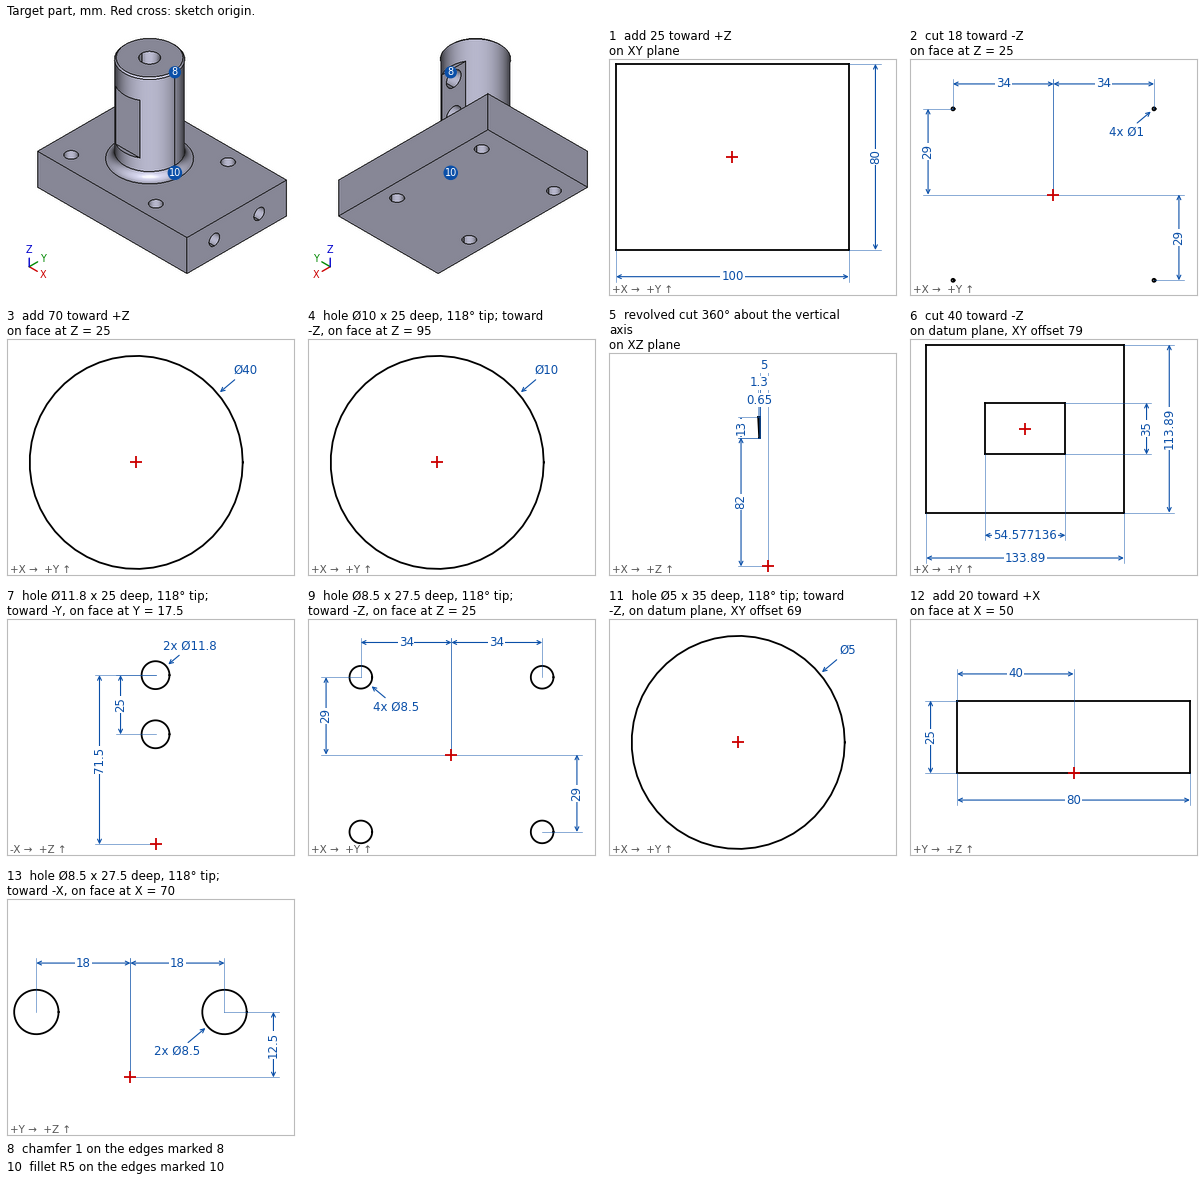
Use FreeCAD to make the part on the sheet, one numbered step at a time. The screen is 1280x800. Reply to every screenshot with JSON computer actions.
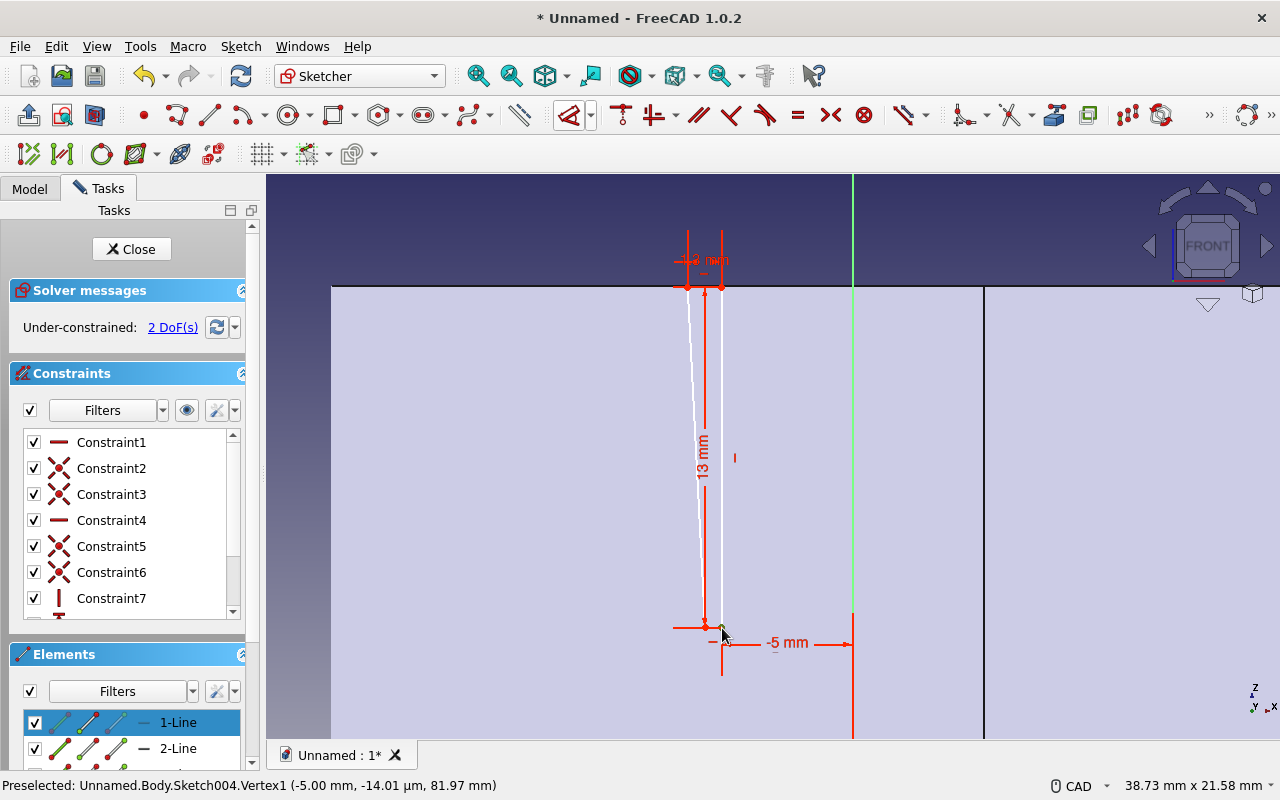
{"action": "key", "text": "i"}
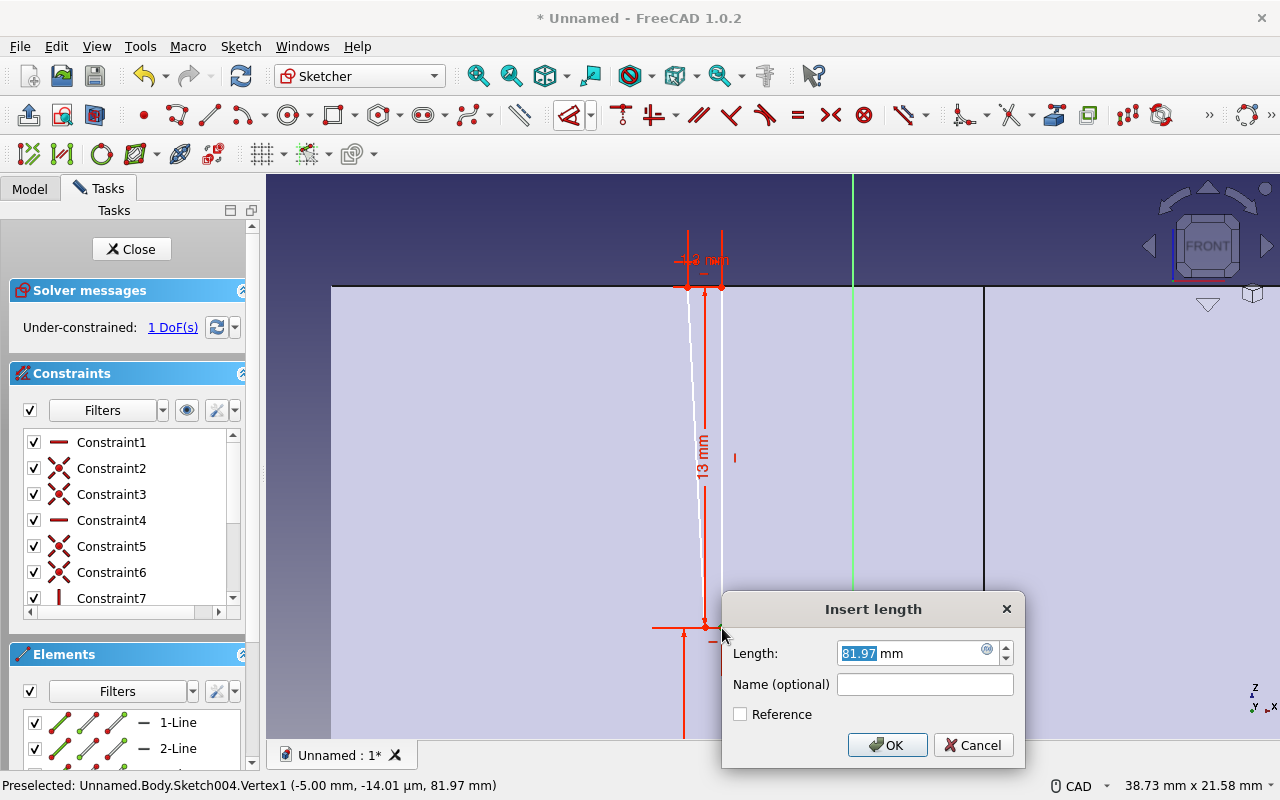
{"action": "type", "text": "82"}
{"action": "key", "text": "Return"}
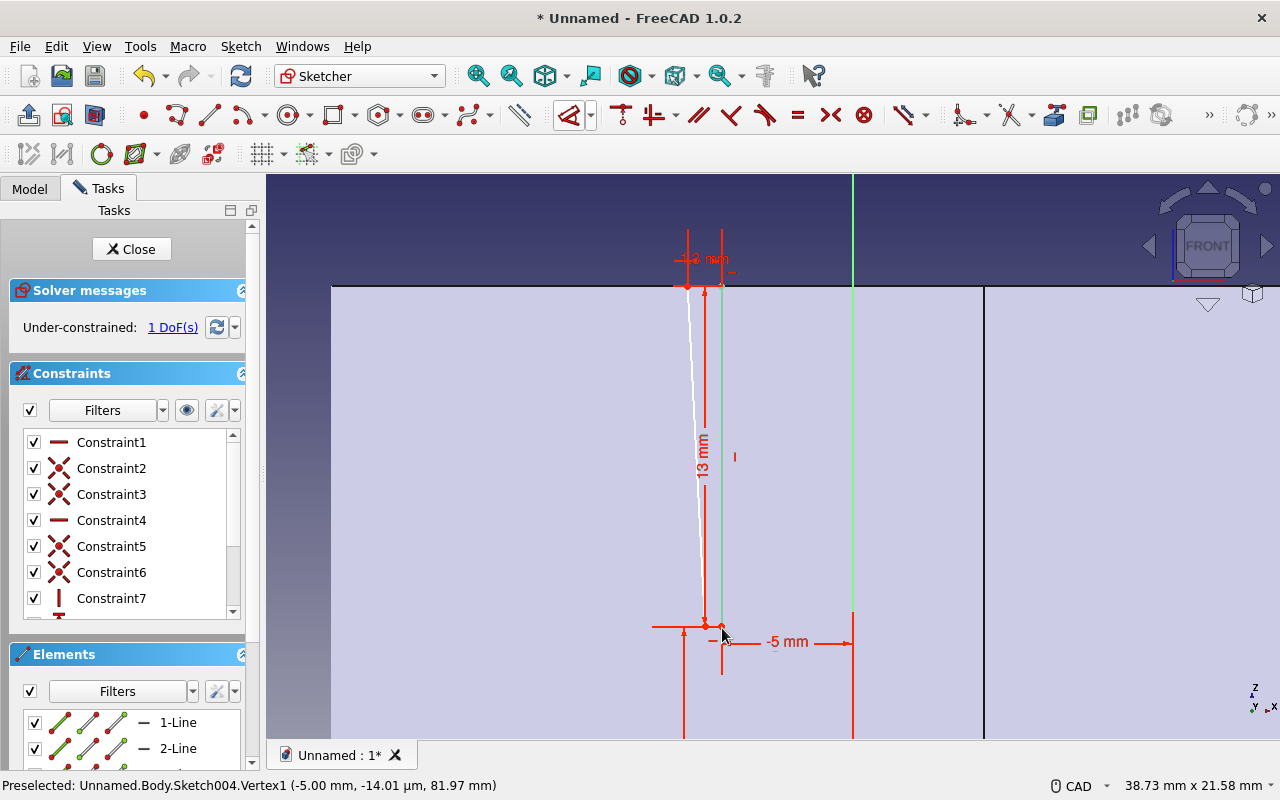
{"action": "scroll", "coordinate": [713, 627], "scroll_direction": "up", "scroll_amount": 5}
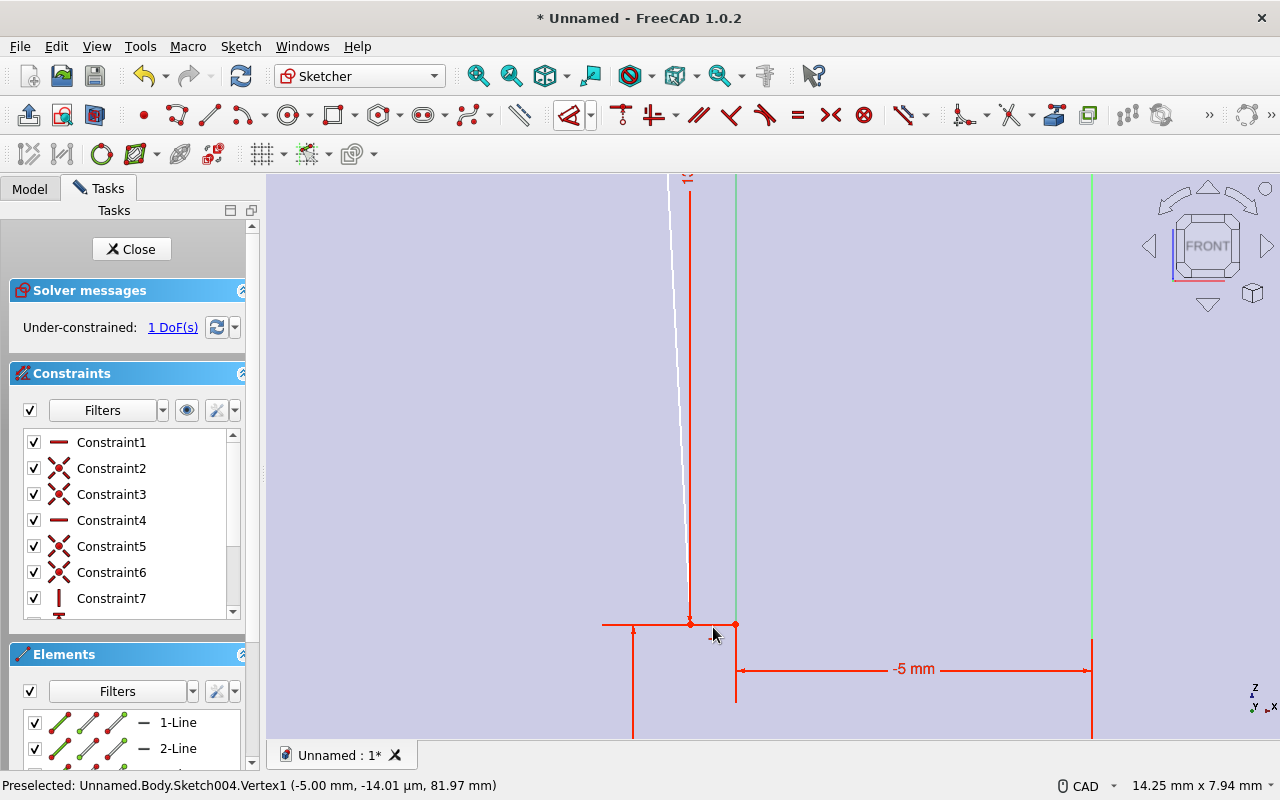
{"action": "left_click", "coordinate": [713, 625]}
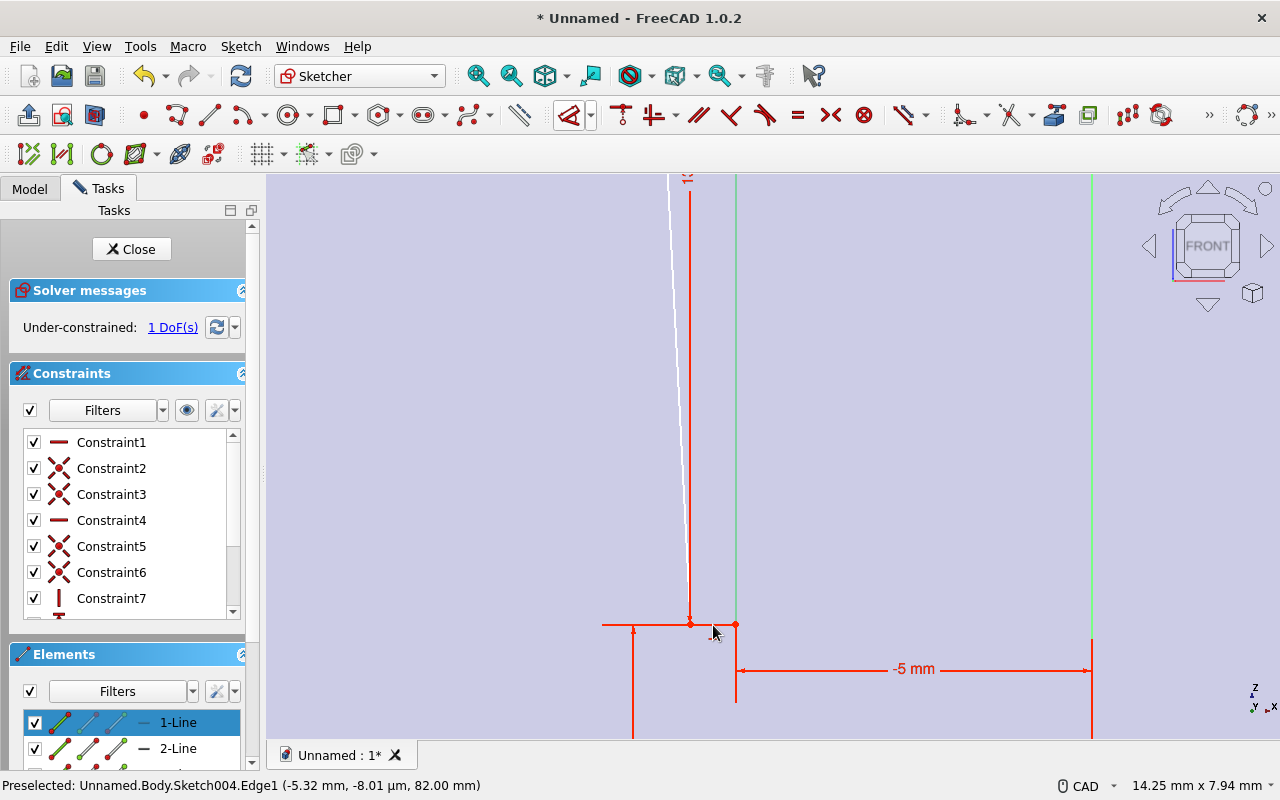
{"action": "left_click", "coordinate": [590, 116]}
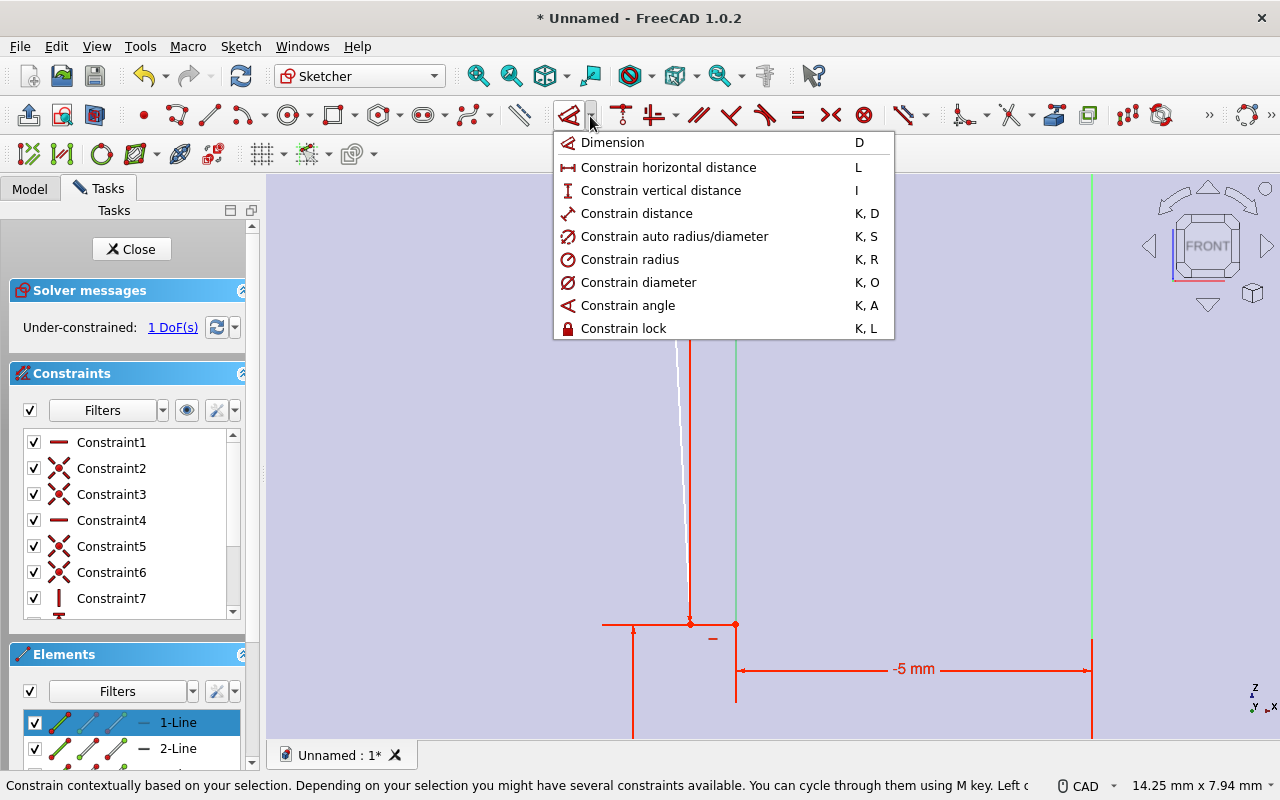
{"action": "left_click", "coordinate": [724, 168]}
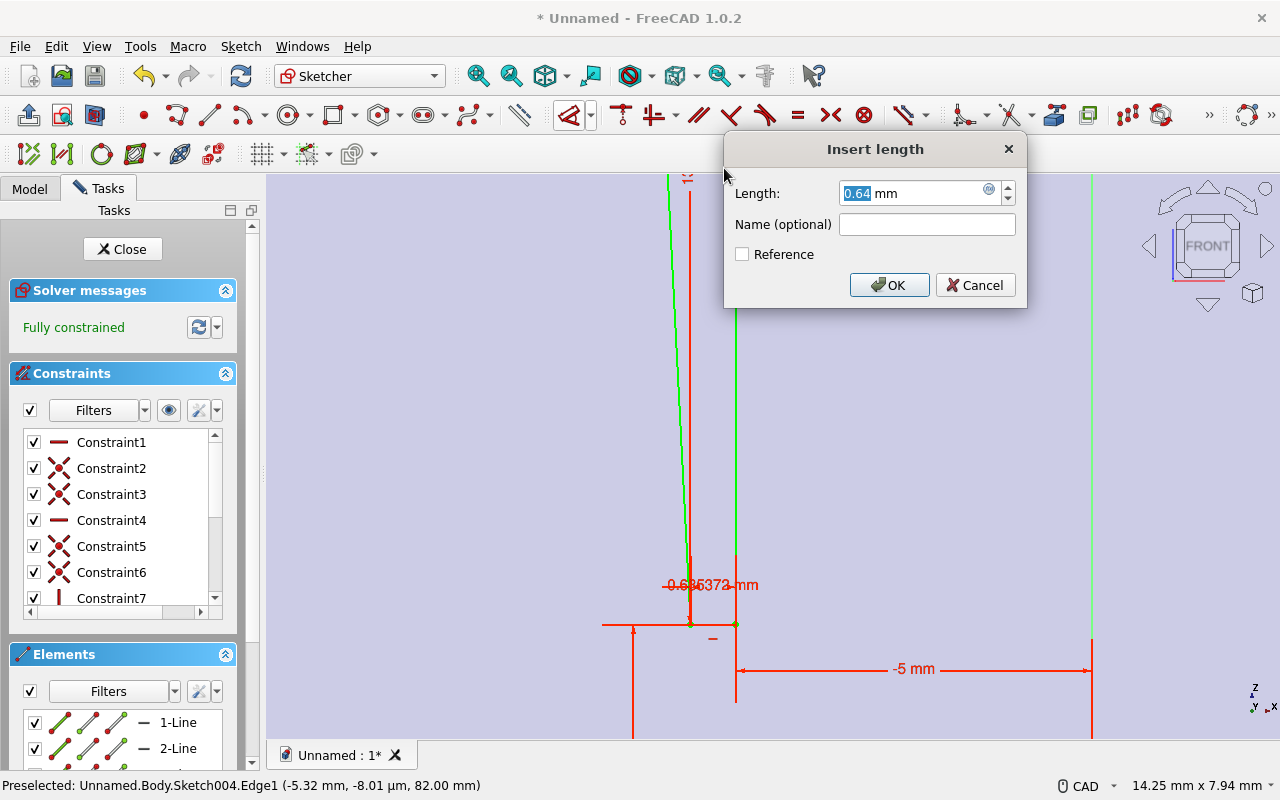
{"action": "type", "text": "0.65"}
{"action": "key", "text": "Return"}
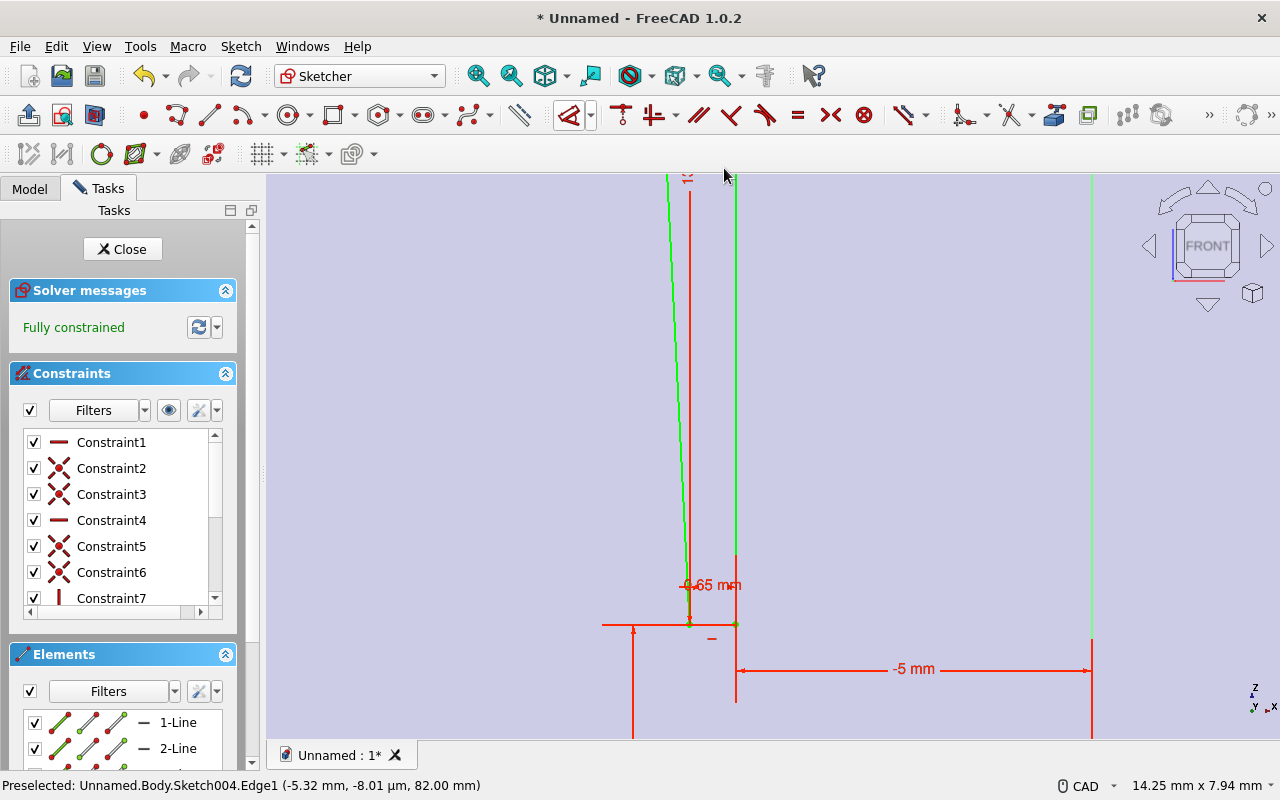
{"action": "left_click", "coordinate": [123, 249]}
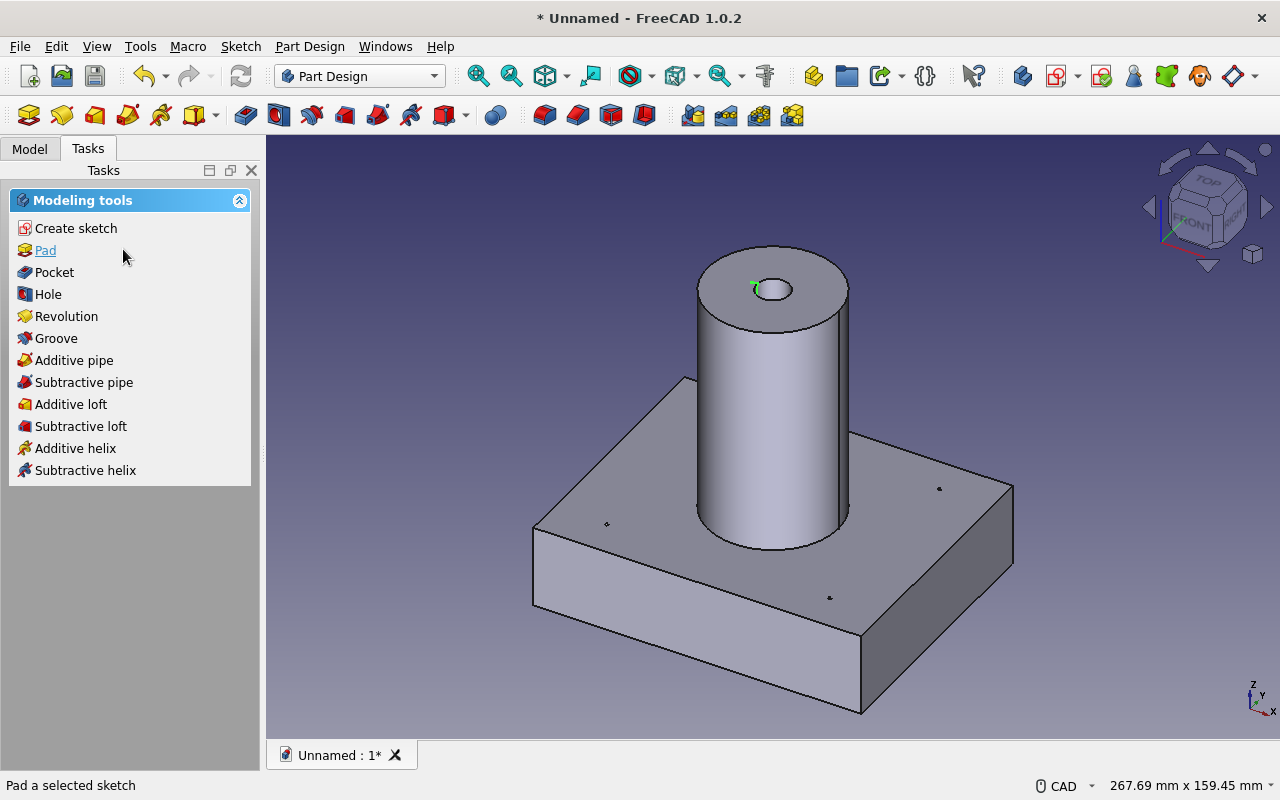
{"action": "left_click", "coordinate": [312, 116]}